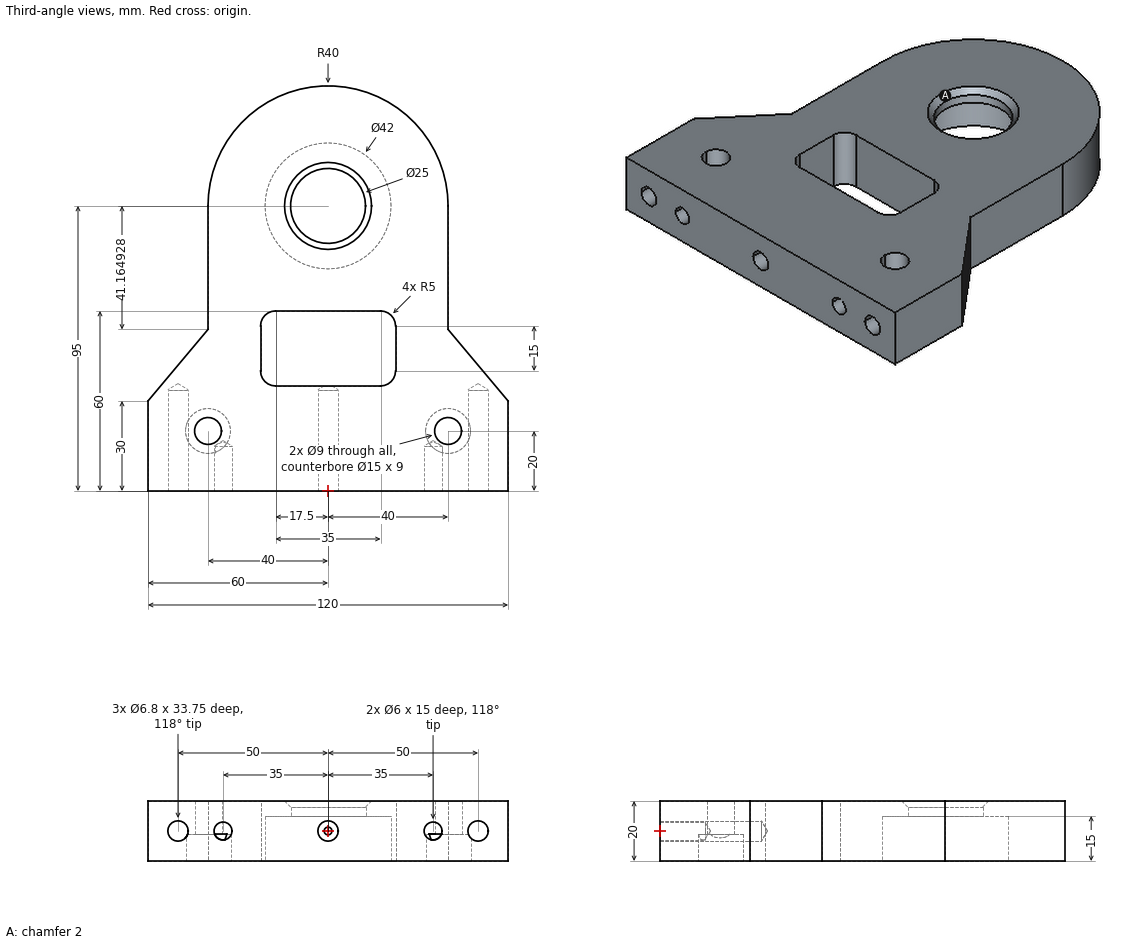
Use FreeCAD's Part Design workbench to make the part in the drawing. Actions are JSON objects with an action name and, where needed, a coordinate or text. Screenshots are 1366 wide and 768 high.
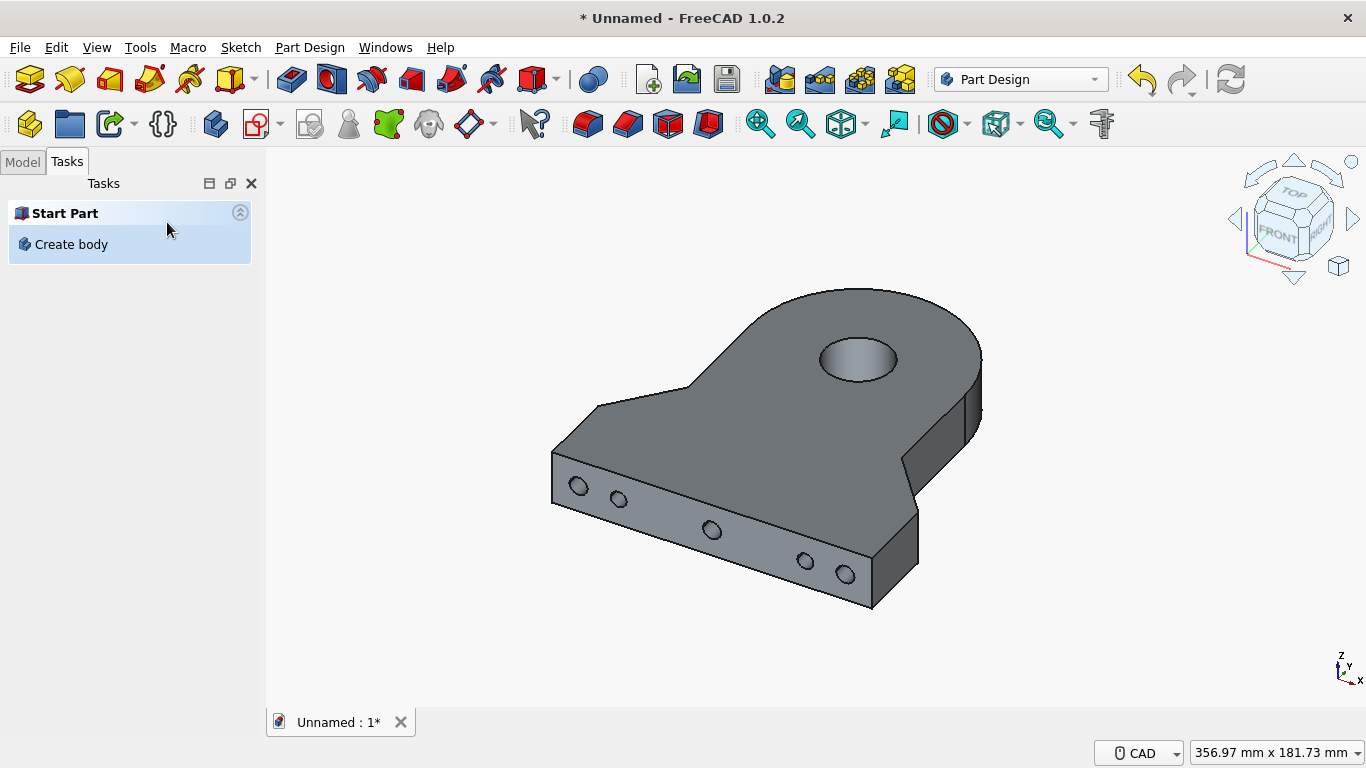
{"action": "key", "text": "5"}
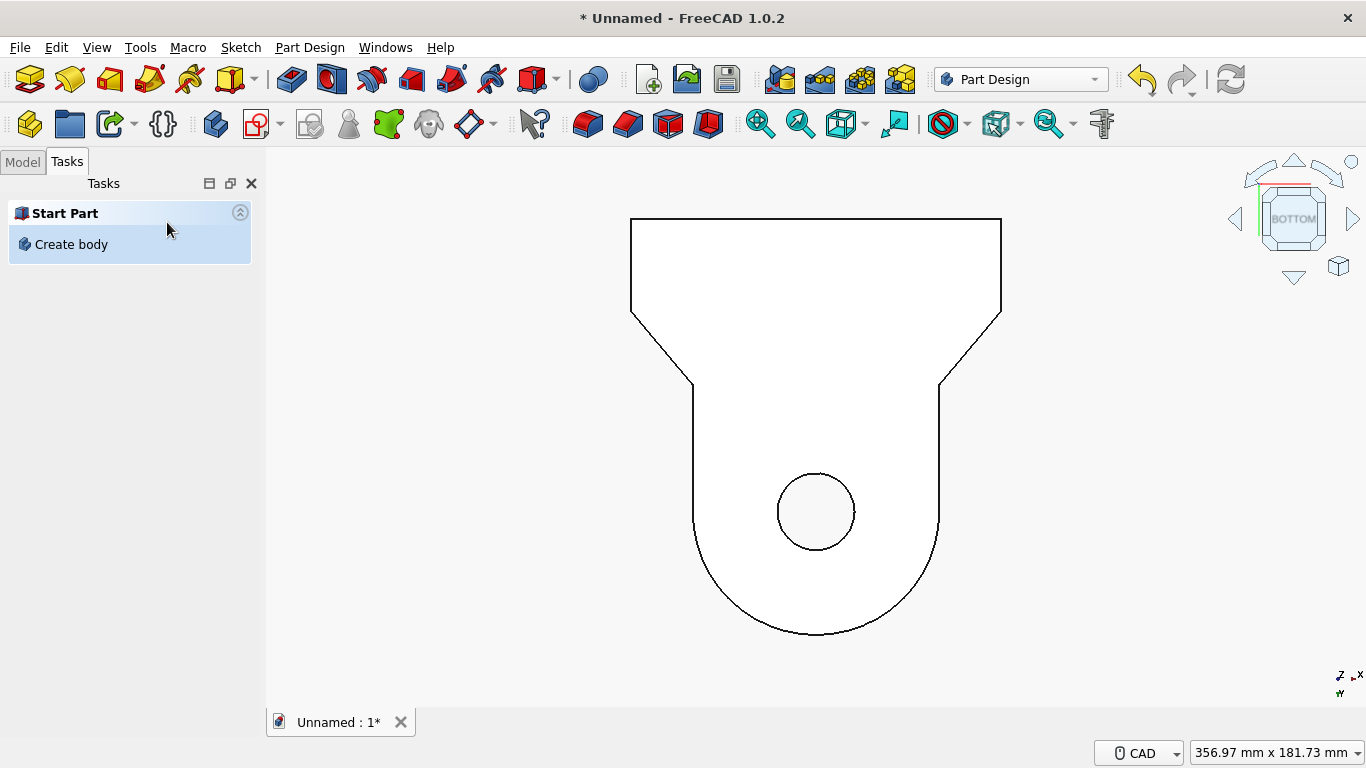
{"action": "left_click", "coordinate": [816, 367]}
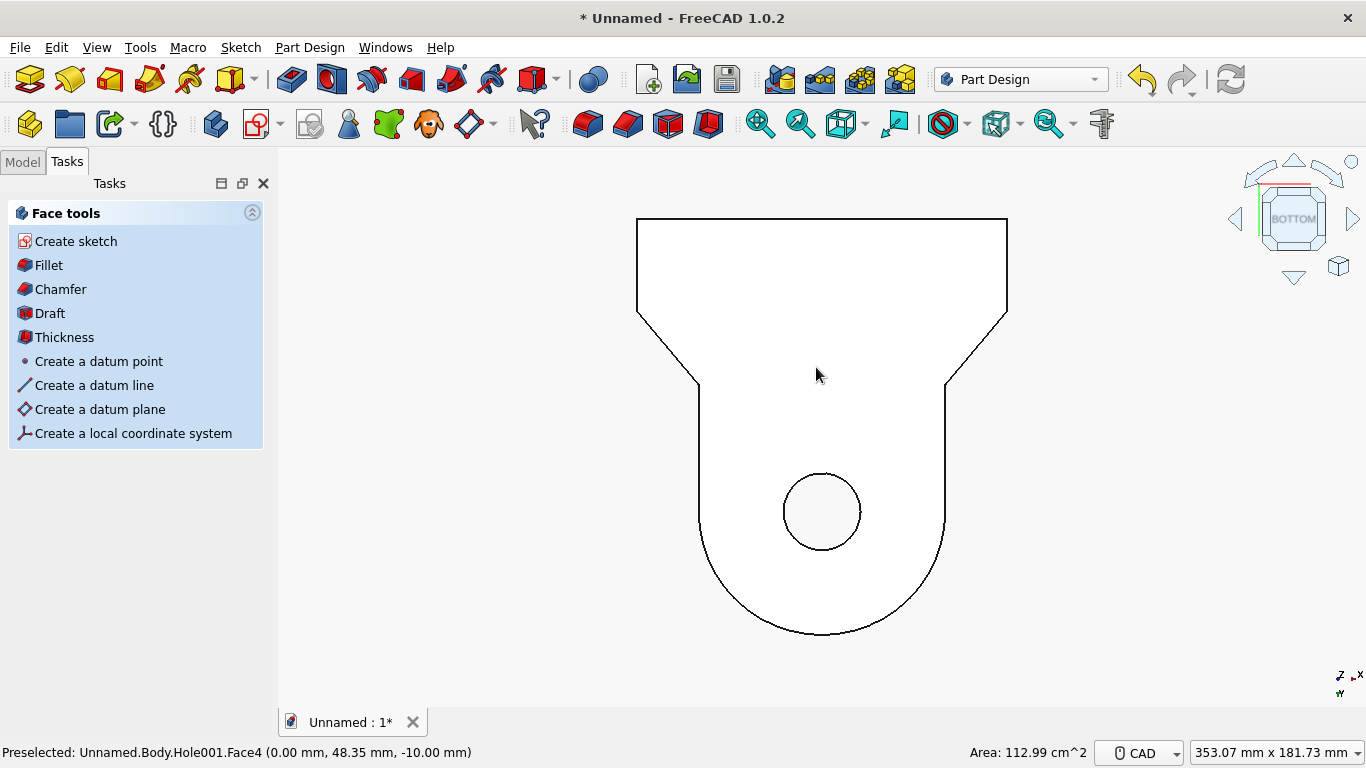
{"action": "left_click", "coordinate": [256, 124]}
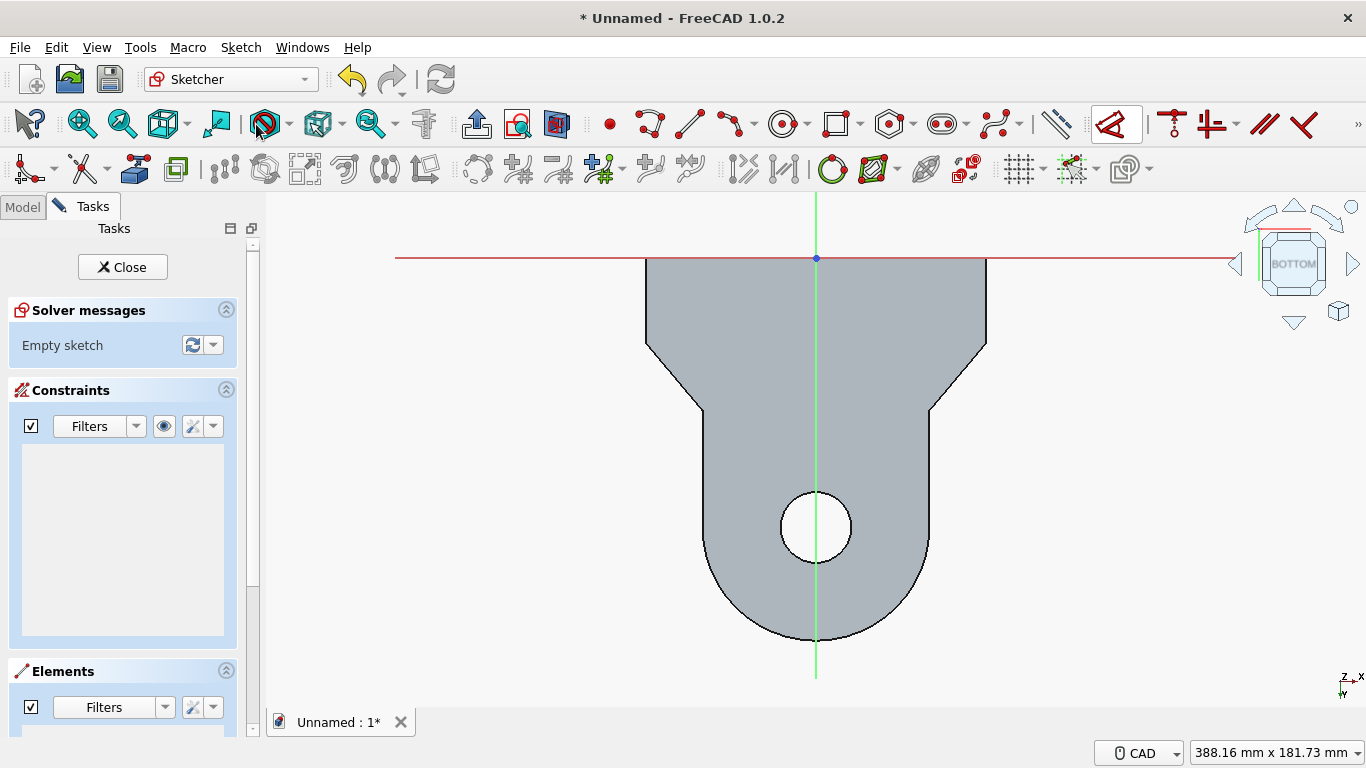
{"action": "scroll", "coordinate": [856, 573], "scroll_direction": "up", "scroll_amount": 5}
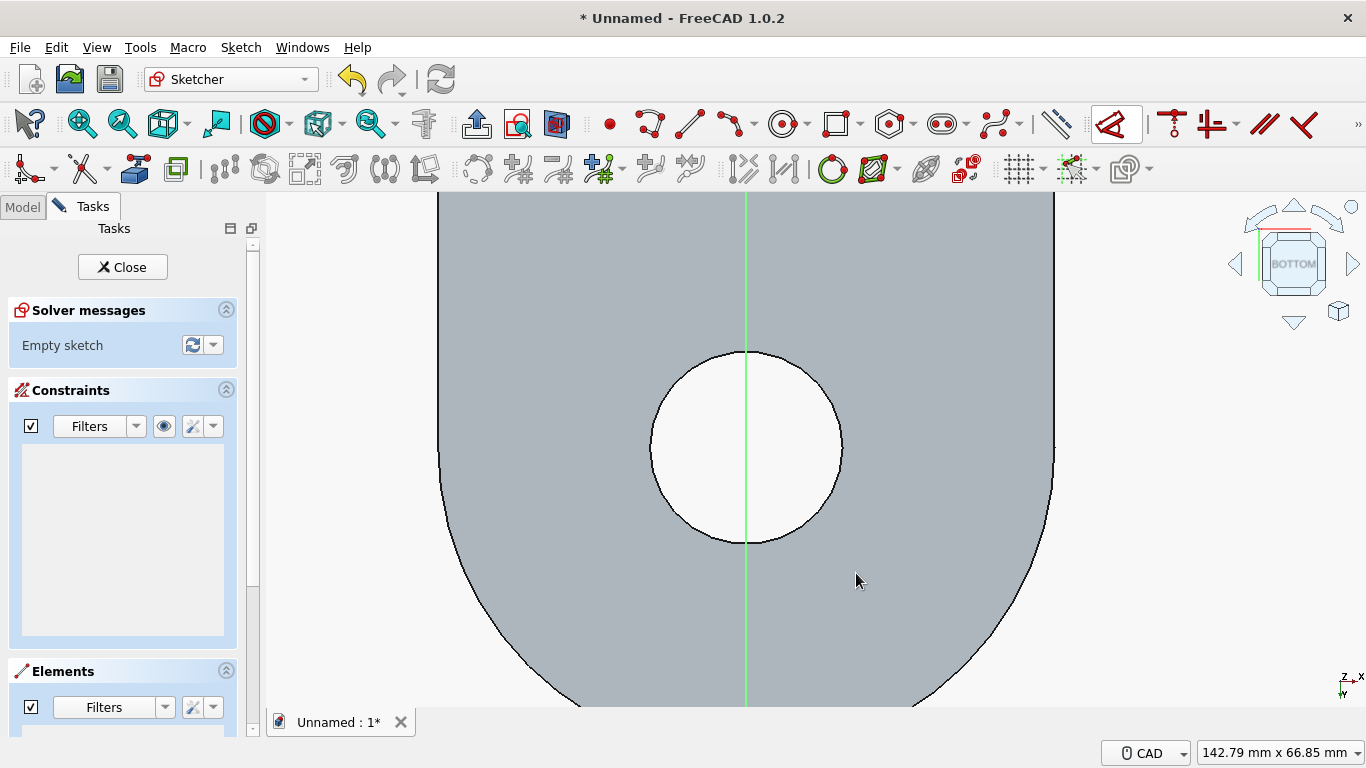
{"action": "left_click", "coordinate": [784, 124]}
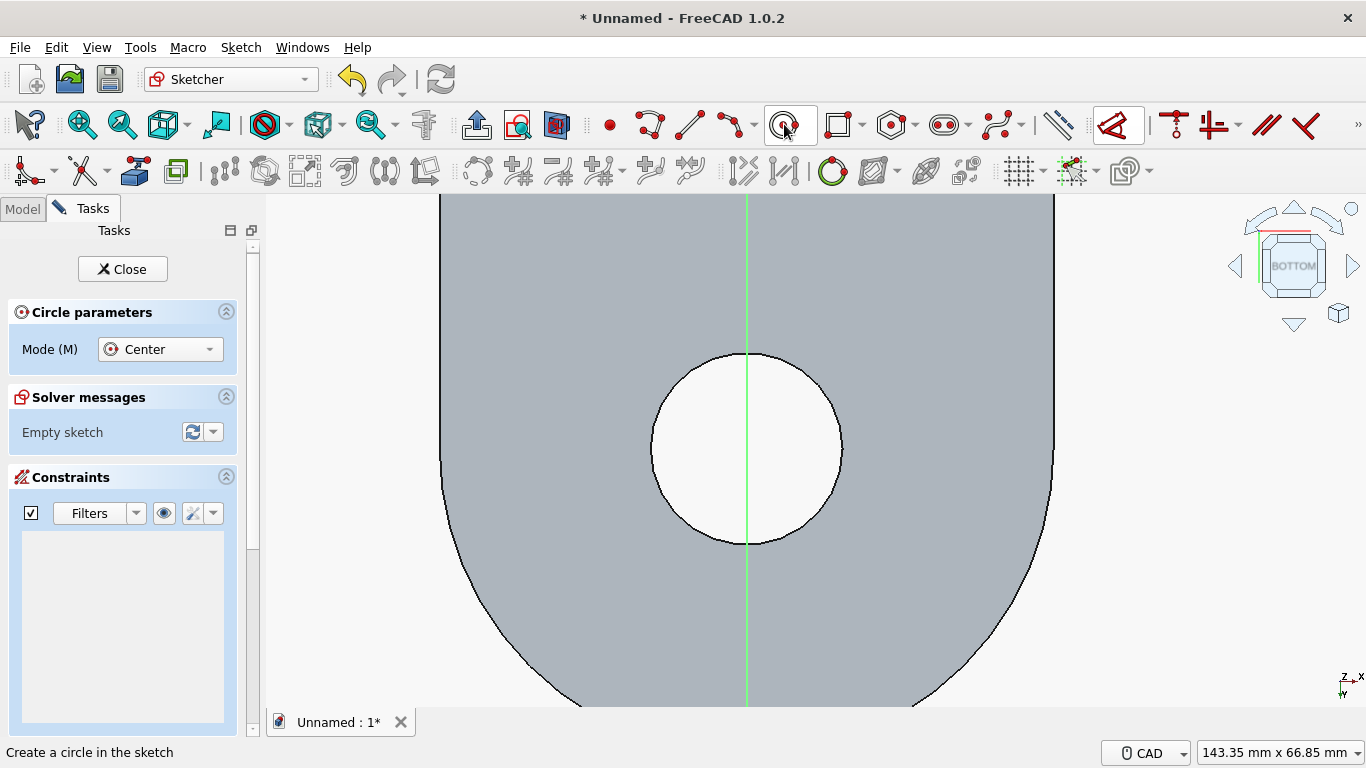
{"action": "left_click", "coordinate": [747, 449]}
{"action": "left_click", "coordinate": [861, 335]}
{"action": "key", "text": "Escape"}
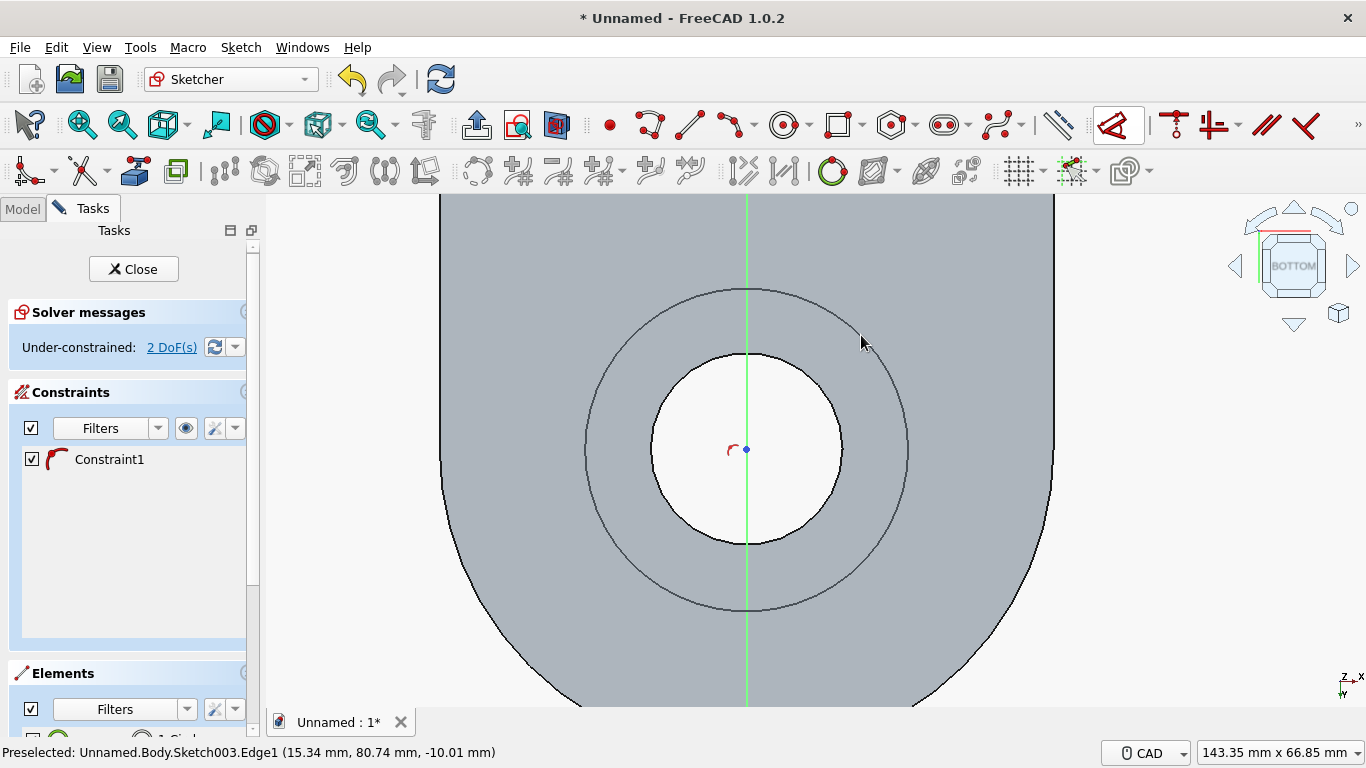
{"action": "left_click", "coordinate": [860, 335]}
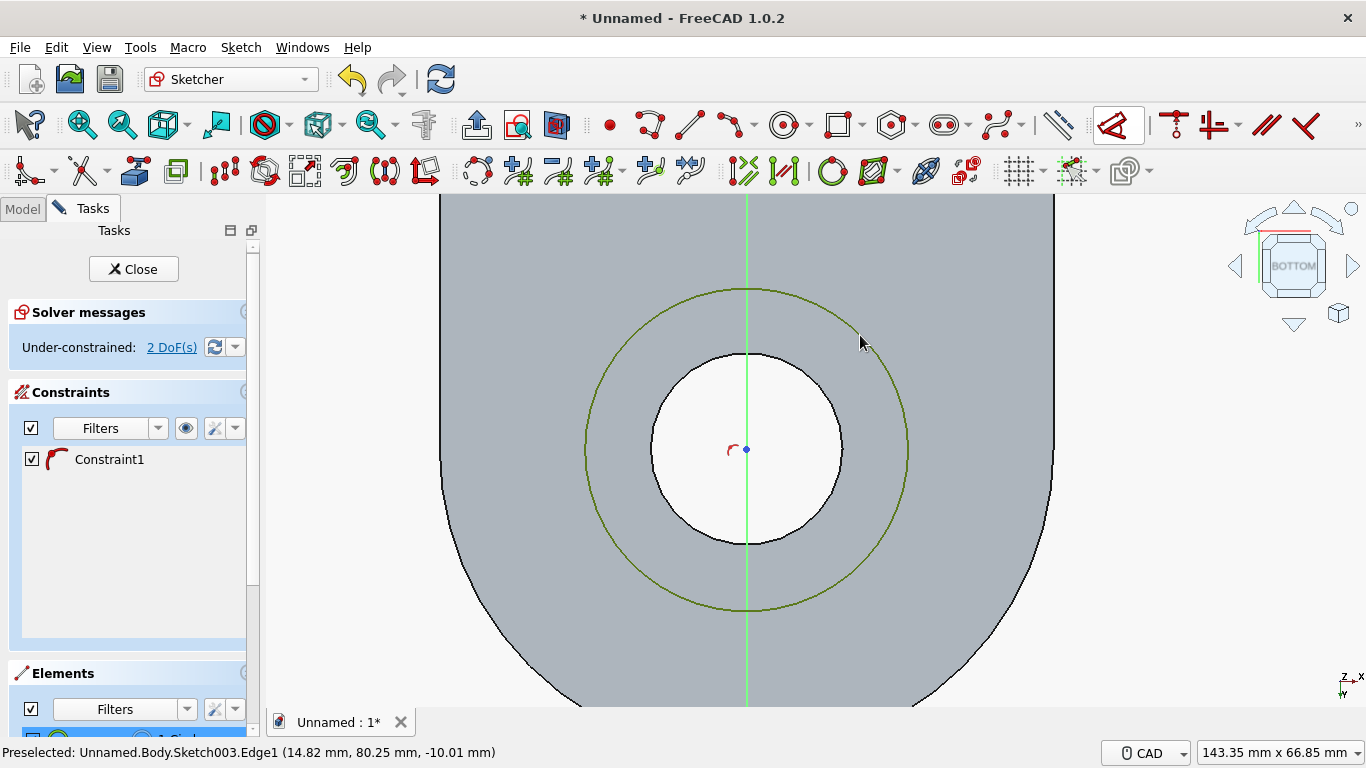
{"action": "key", "text": "k o"}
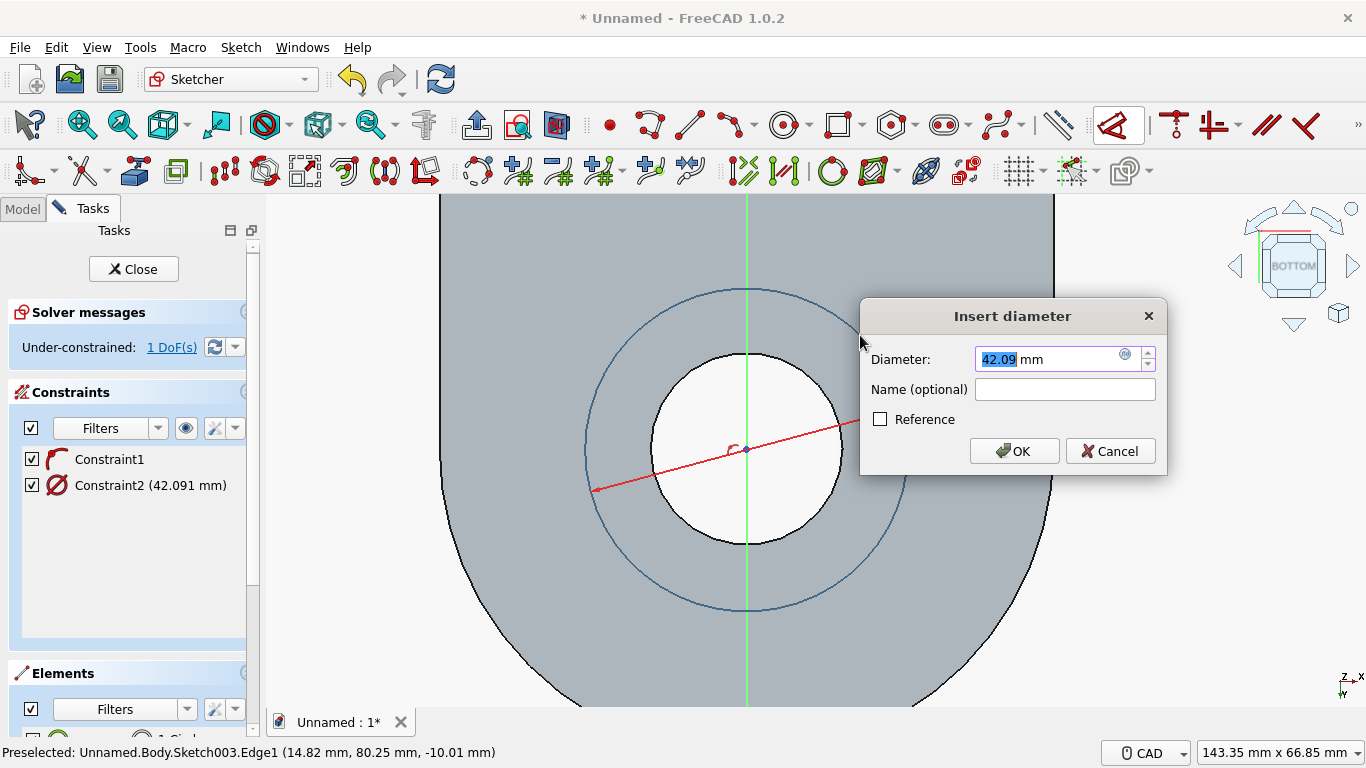
{"action": "type", "text": "42"}
{"action": "key", "text": "Return"}